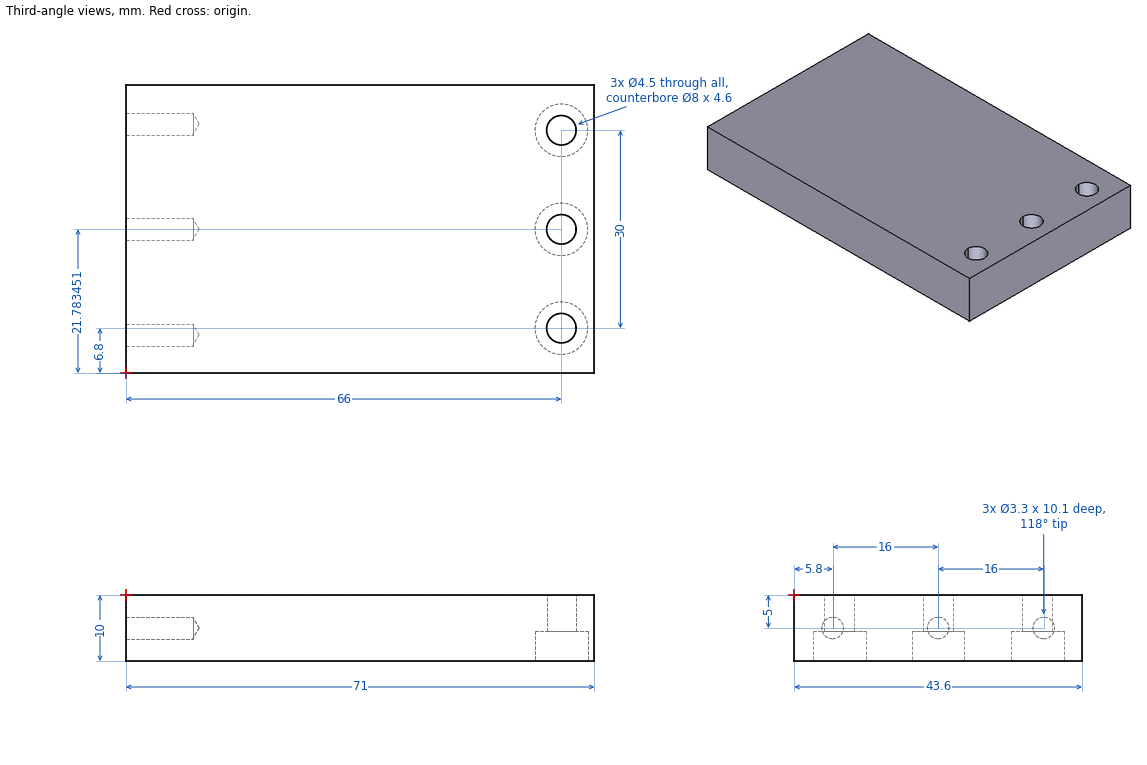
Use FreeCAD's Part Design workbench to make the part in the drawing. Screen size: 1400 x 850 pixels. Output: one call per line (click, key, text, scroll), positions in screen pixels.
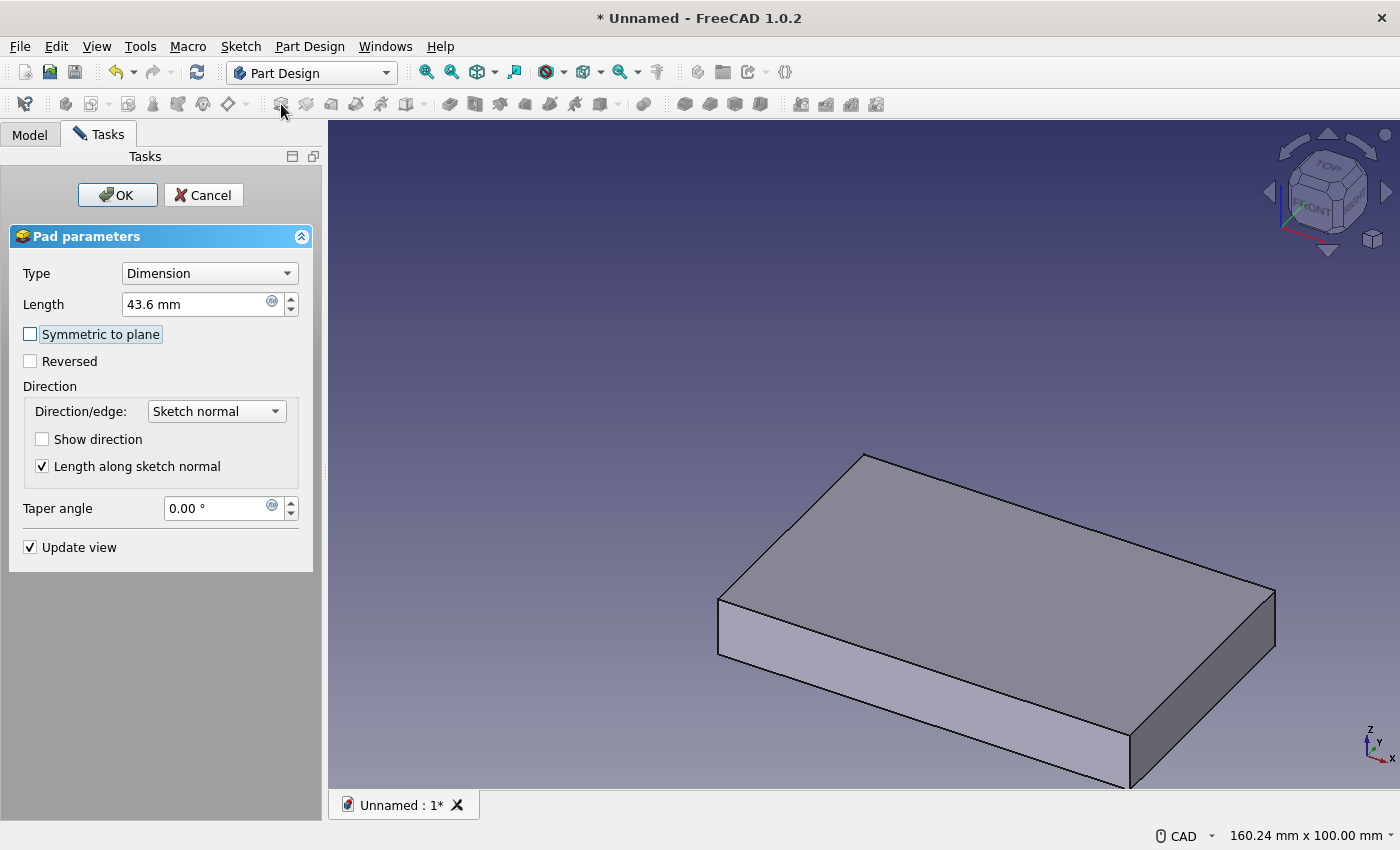
click(31, 361)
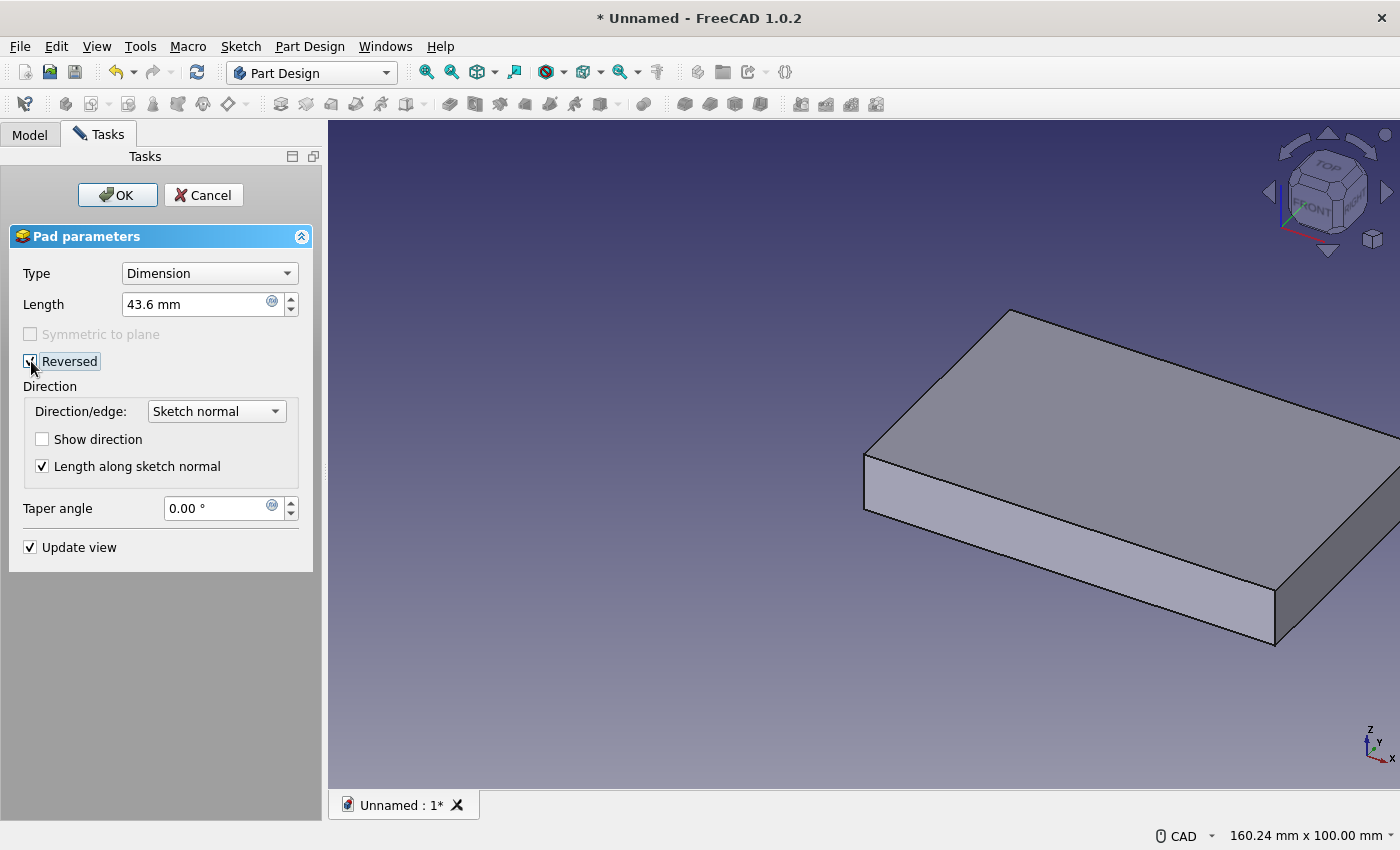
click(118, 195)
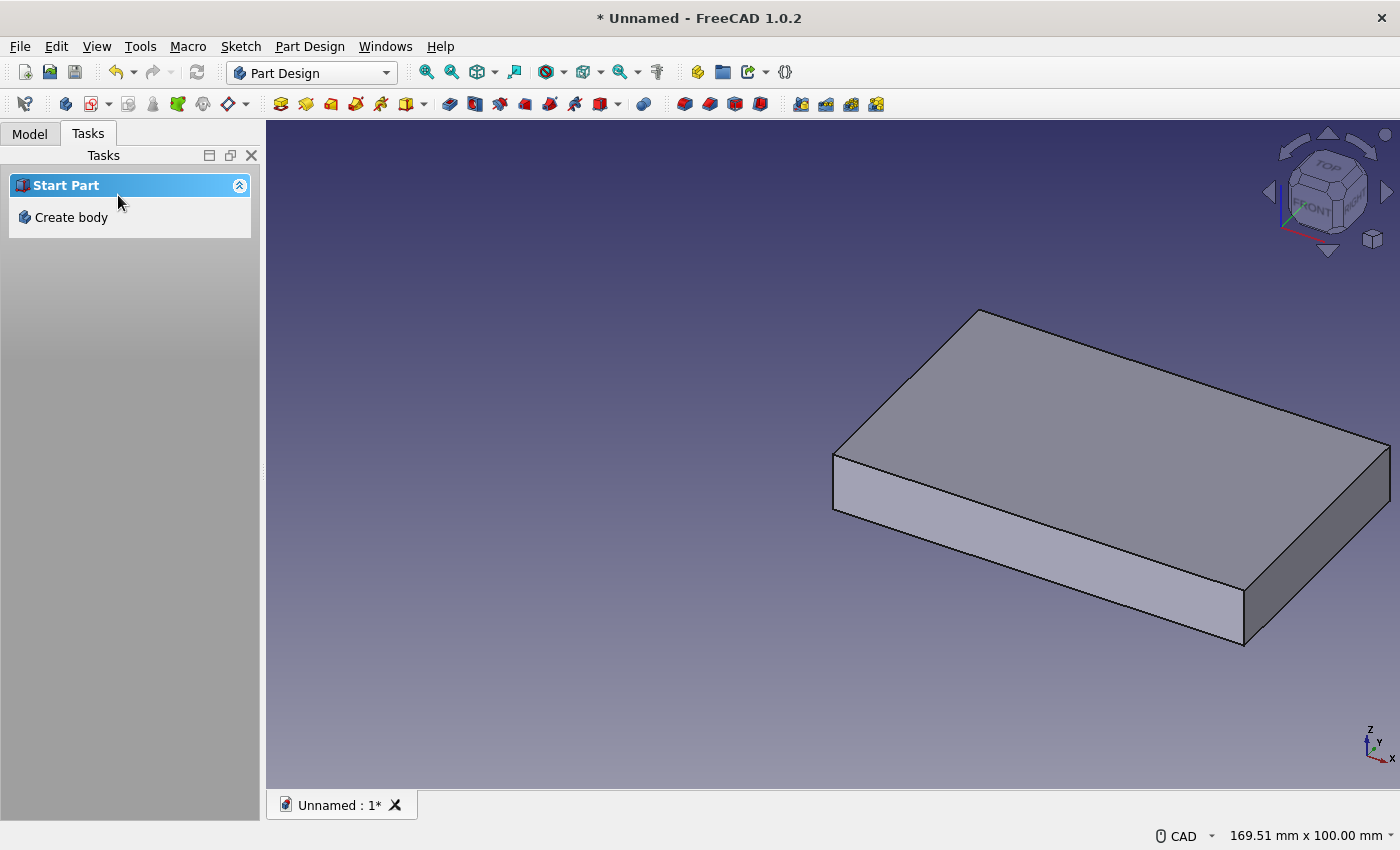
key(5)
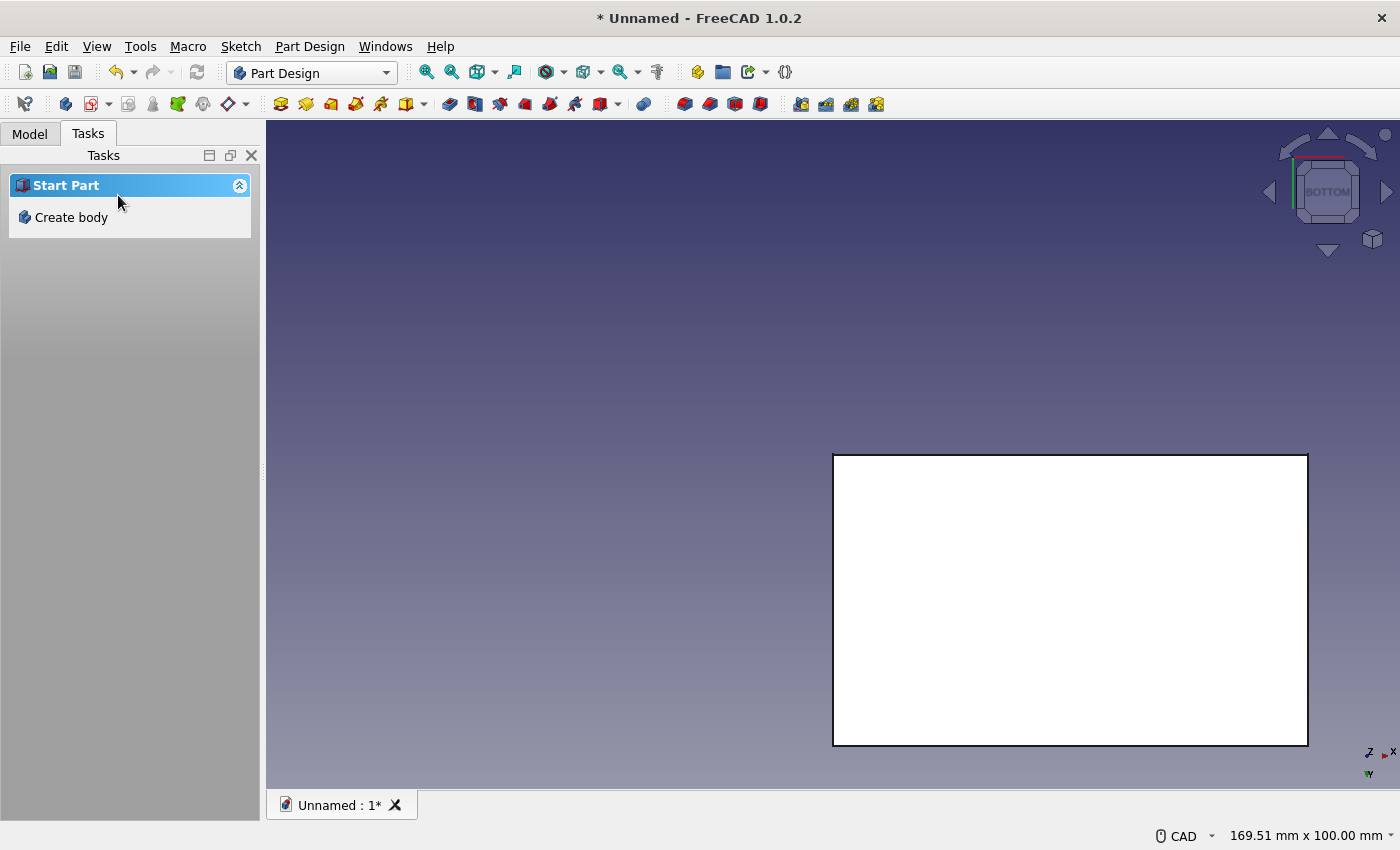
key(v)
key(f)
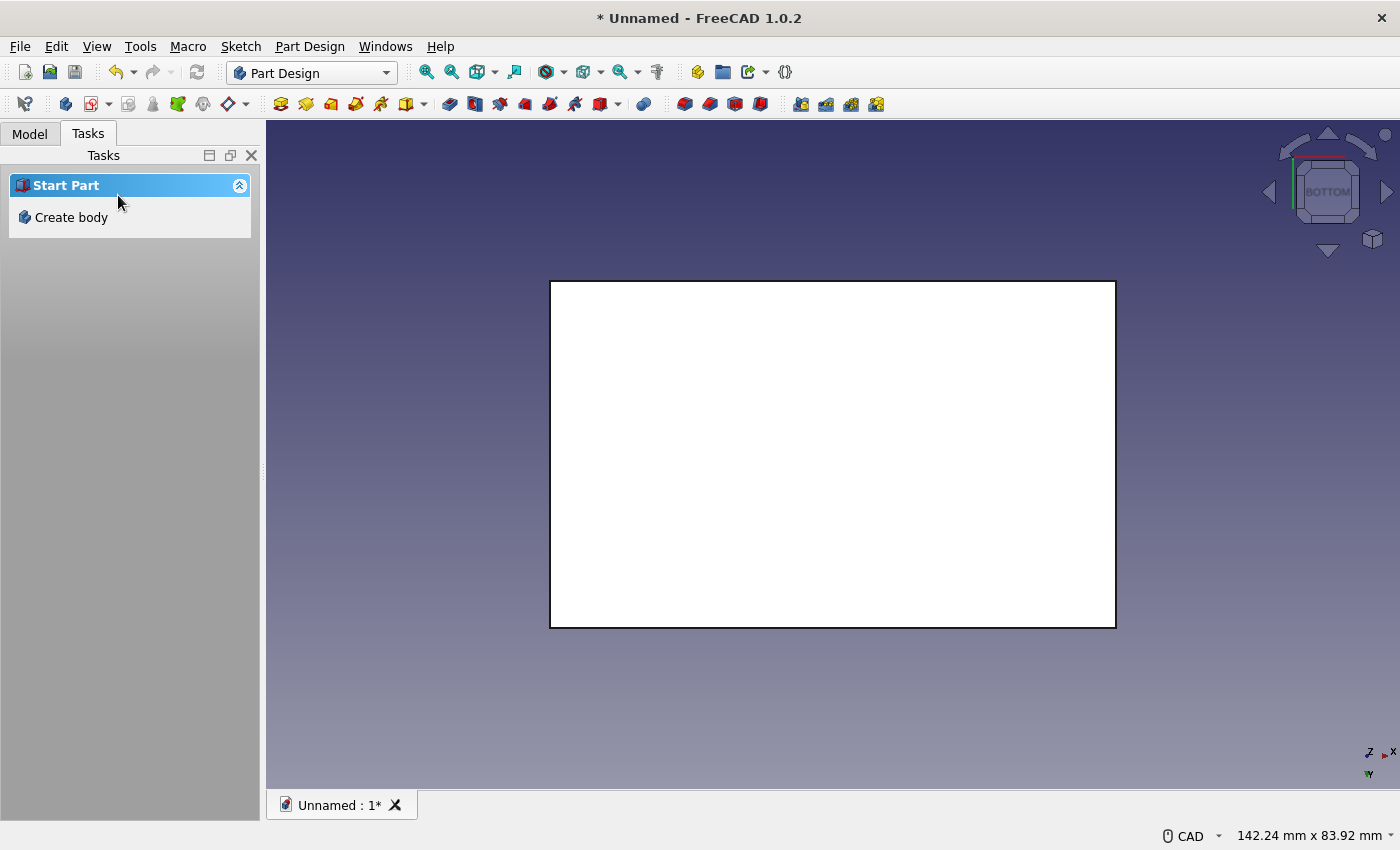
click(914, 453)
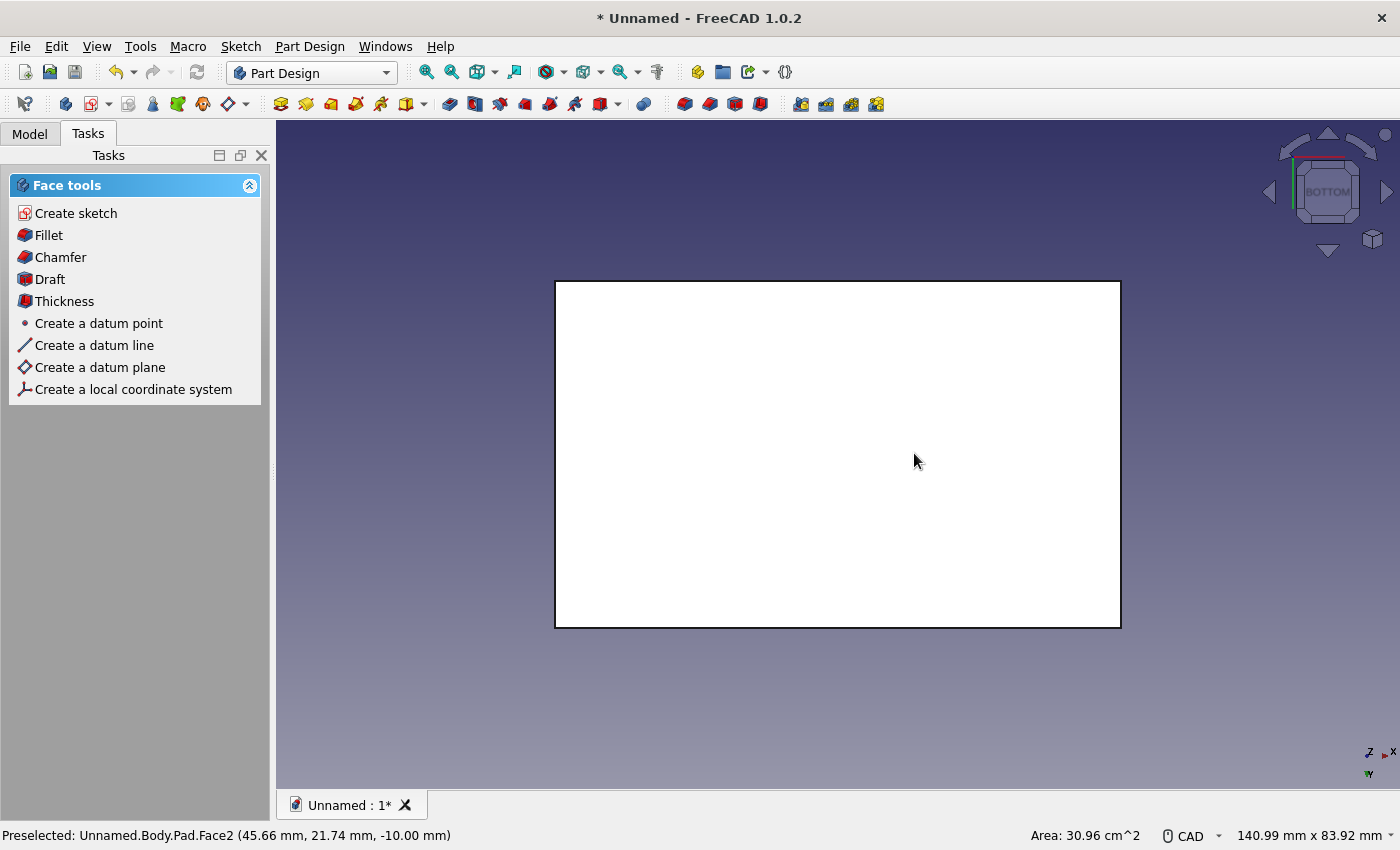
click(90, 104)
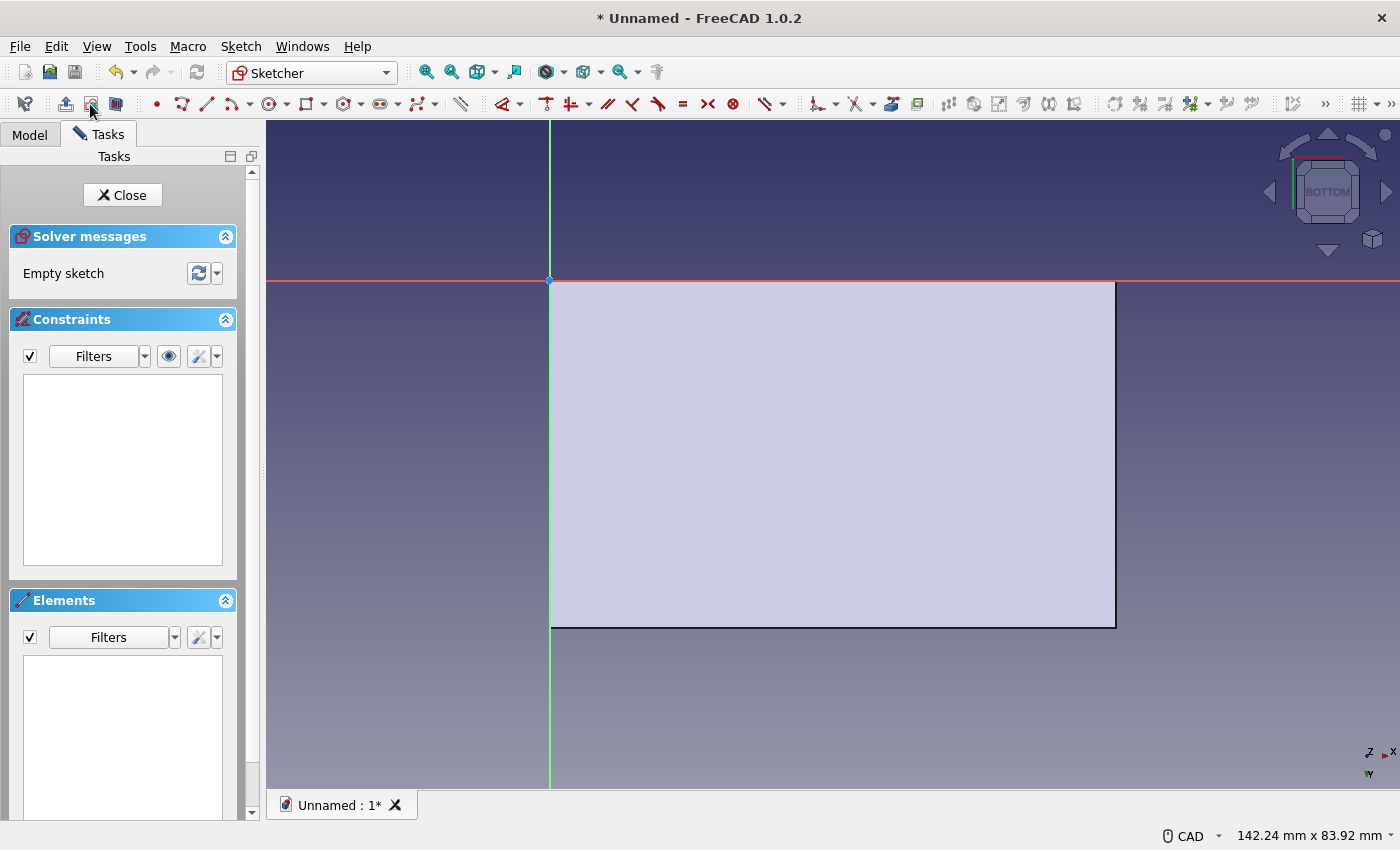
key(g)
key(c)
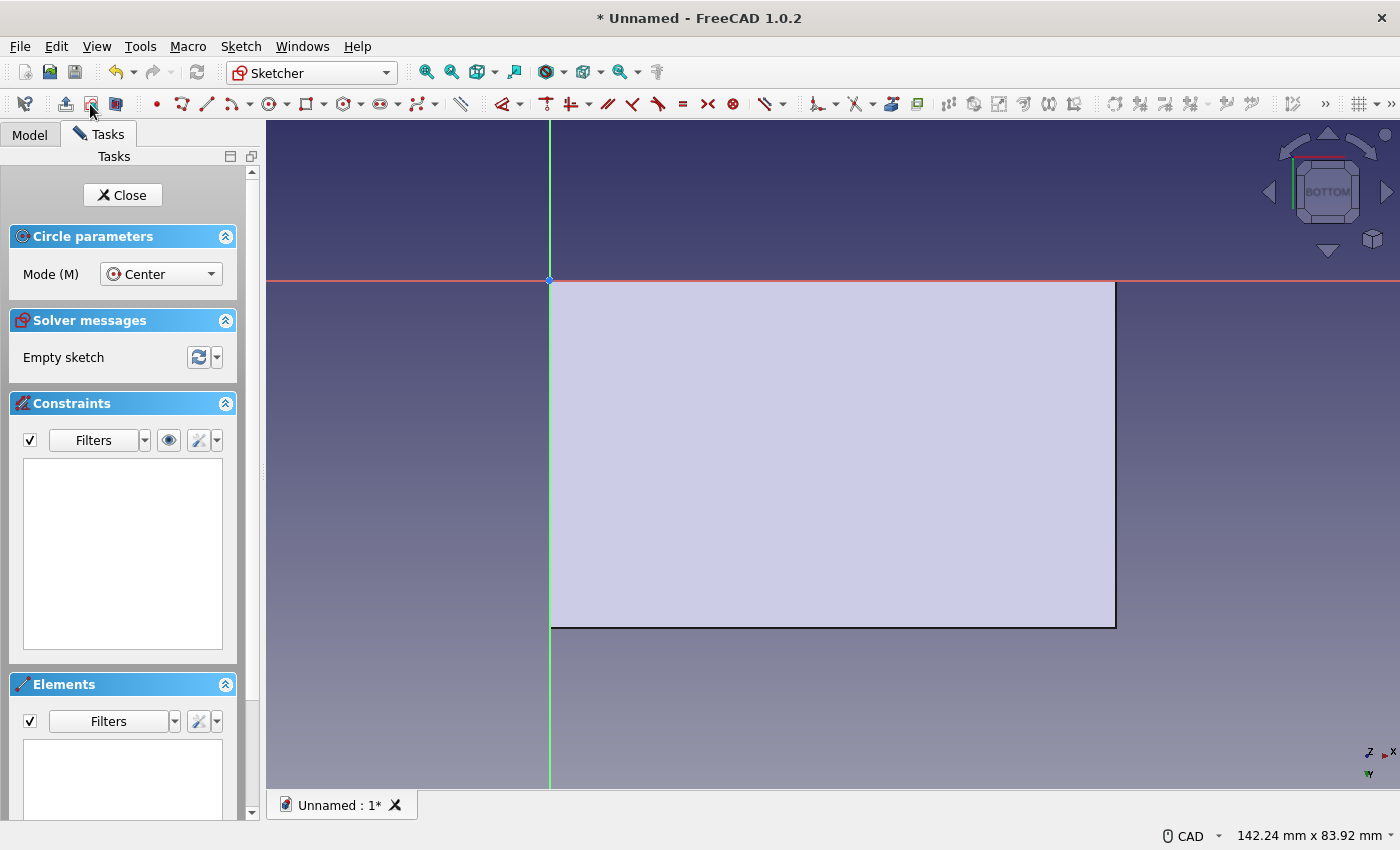
scroll(1076, 574, up, 2)